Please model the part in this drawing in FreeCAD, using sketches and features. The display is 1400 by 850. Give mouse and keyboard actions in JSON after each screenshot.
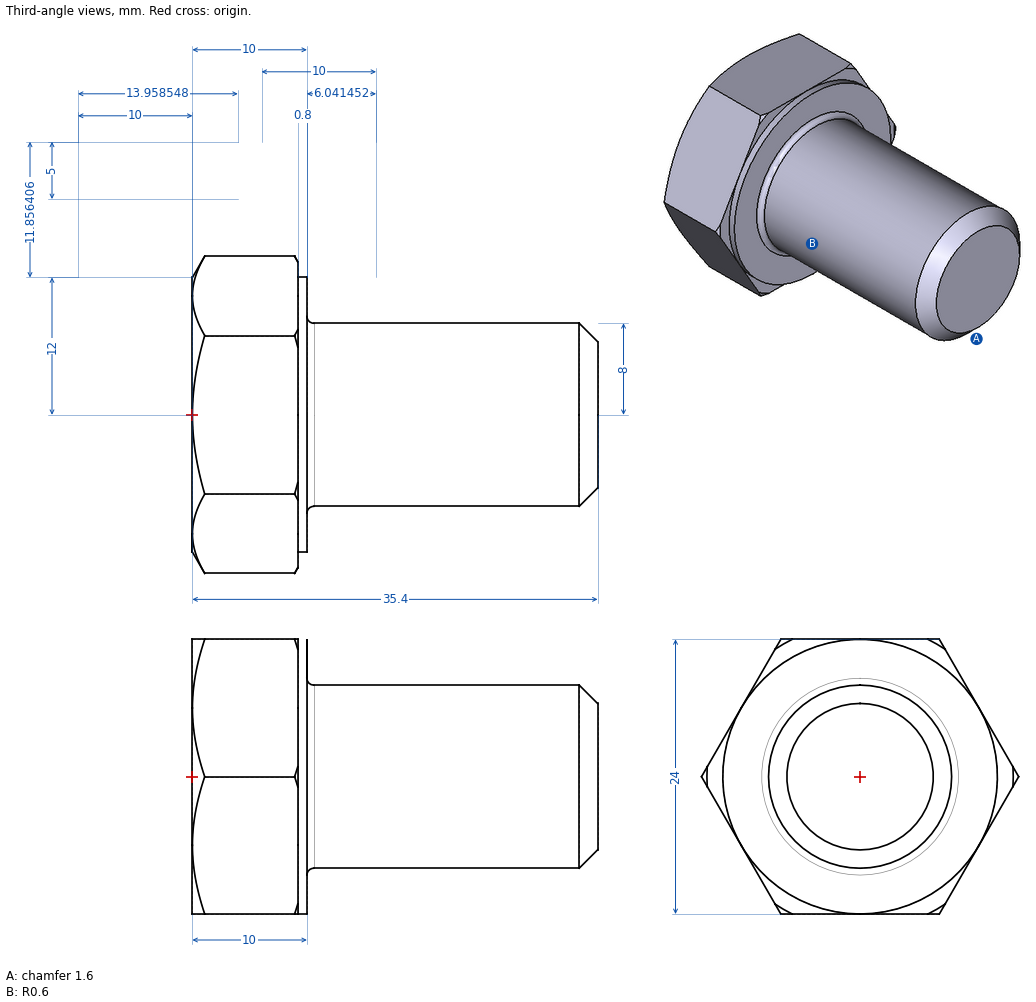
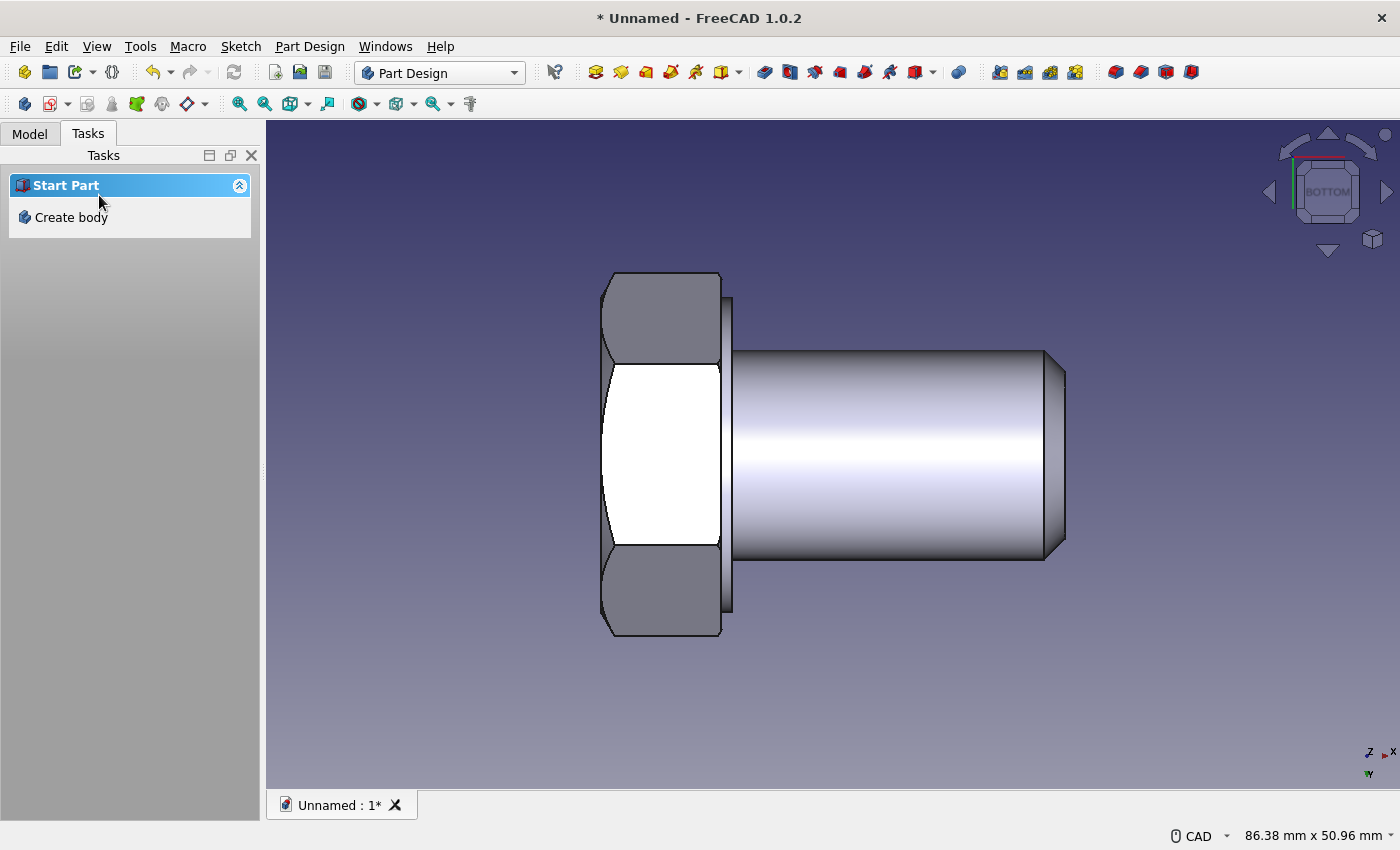
{"action": "key", "text": "4"}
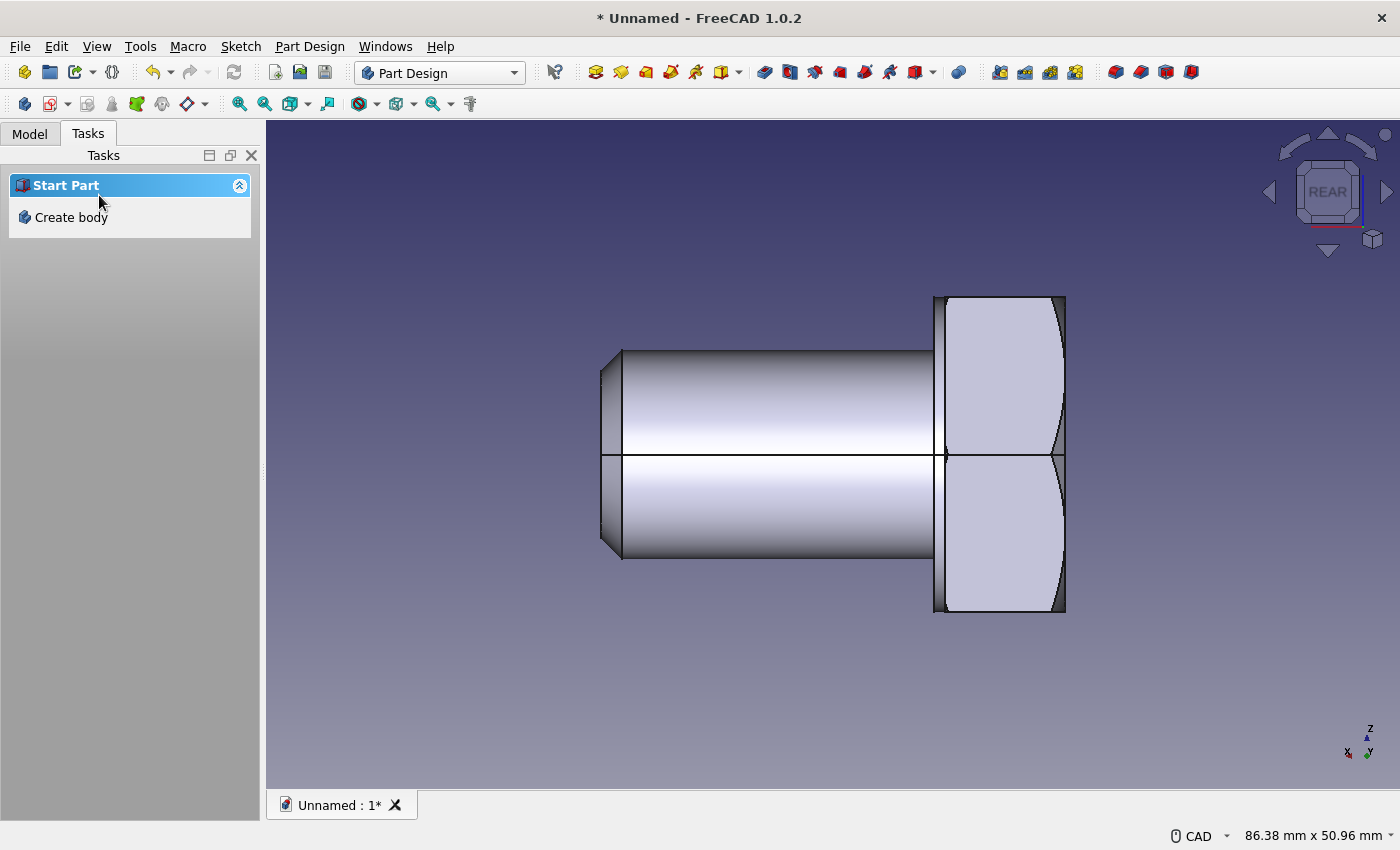
{"action": "key", "text": "6"}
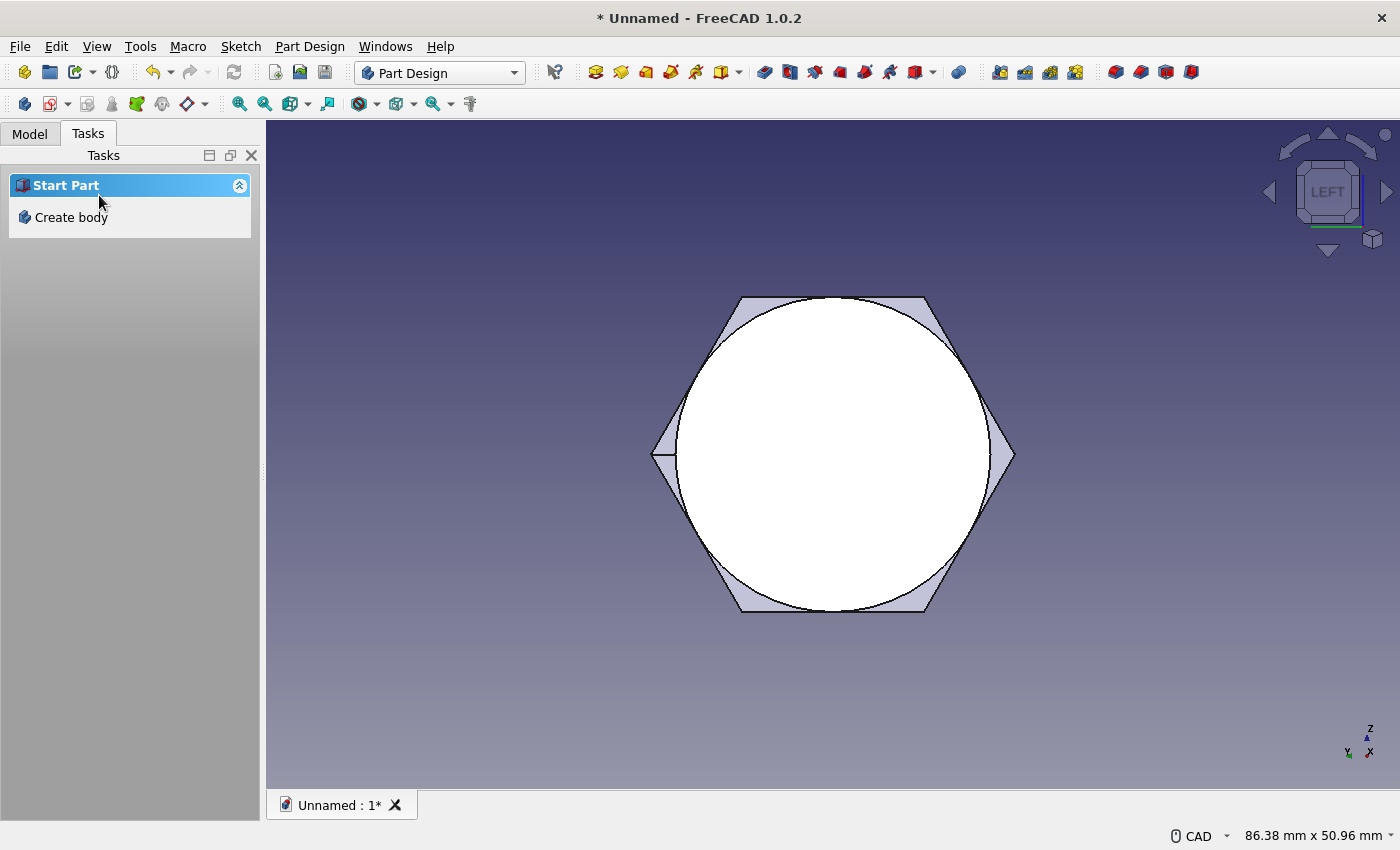
{"action": "key", "text": "v 3"}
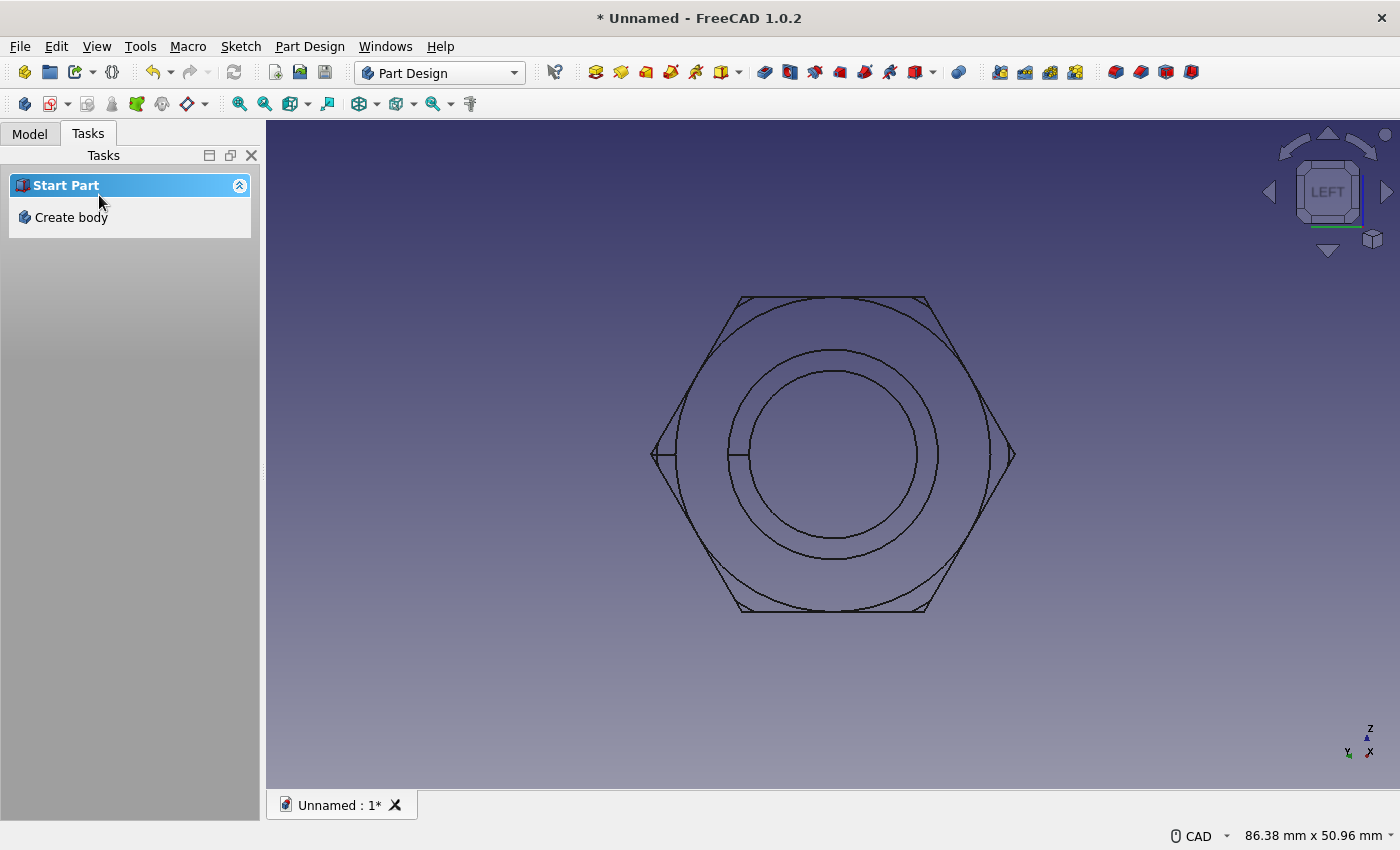
{"action": "key", "text": "0"}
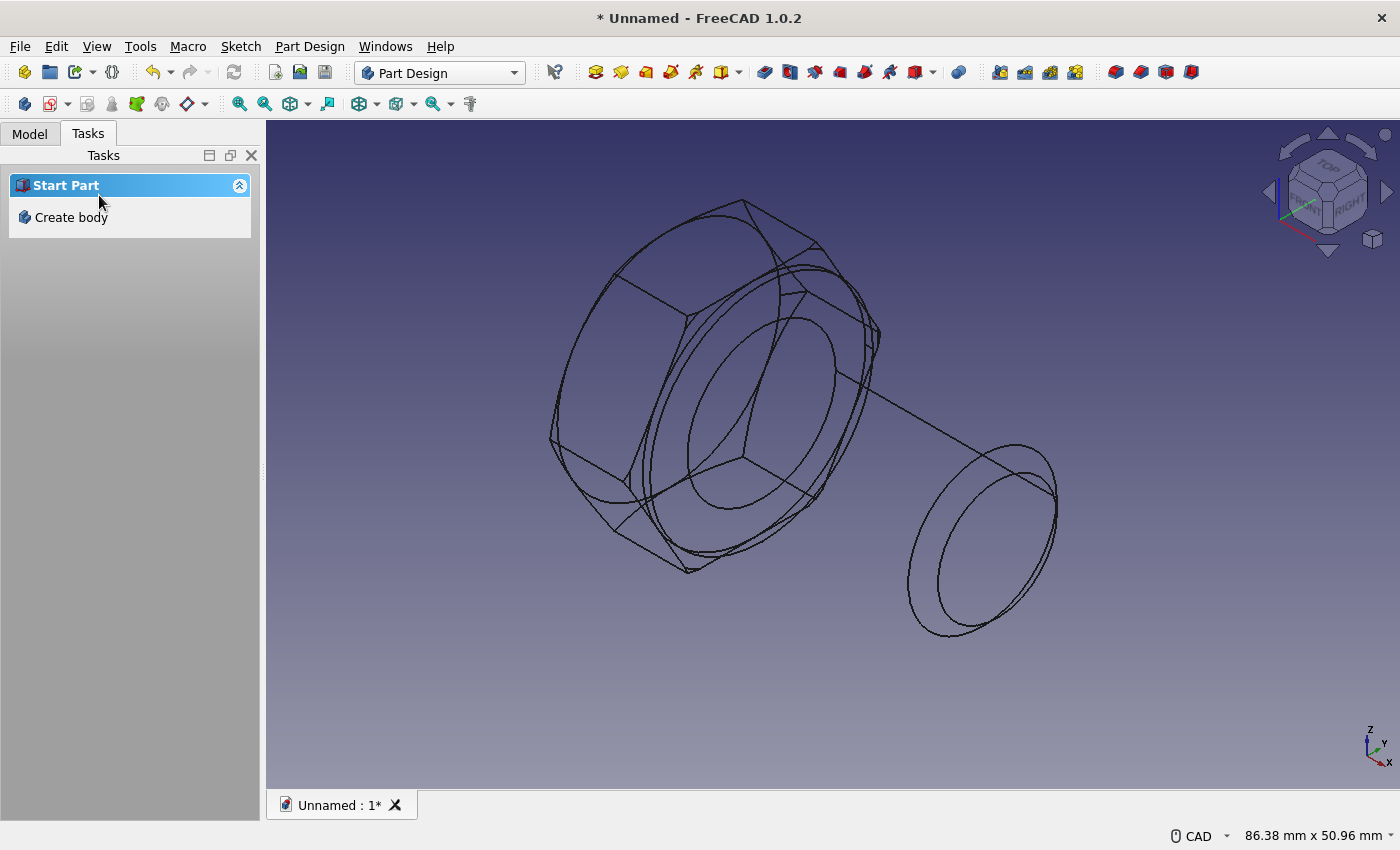
{"action": "left_click", "coordinate": [687, 455]}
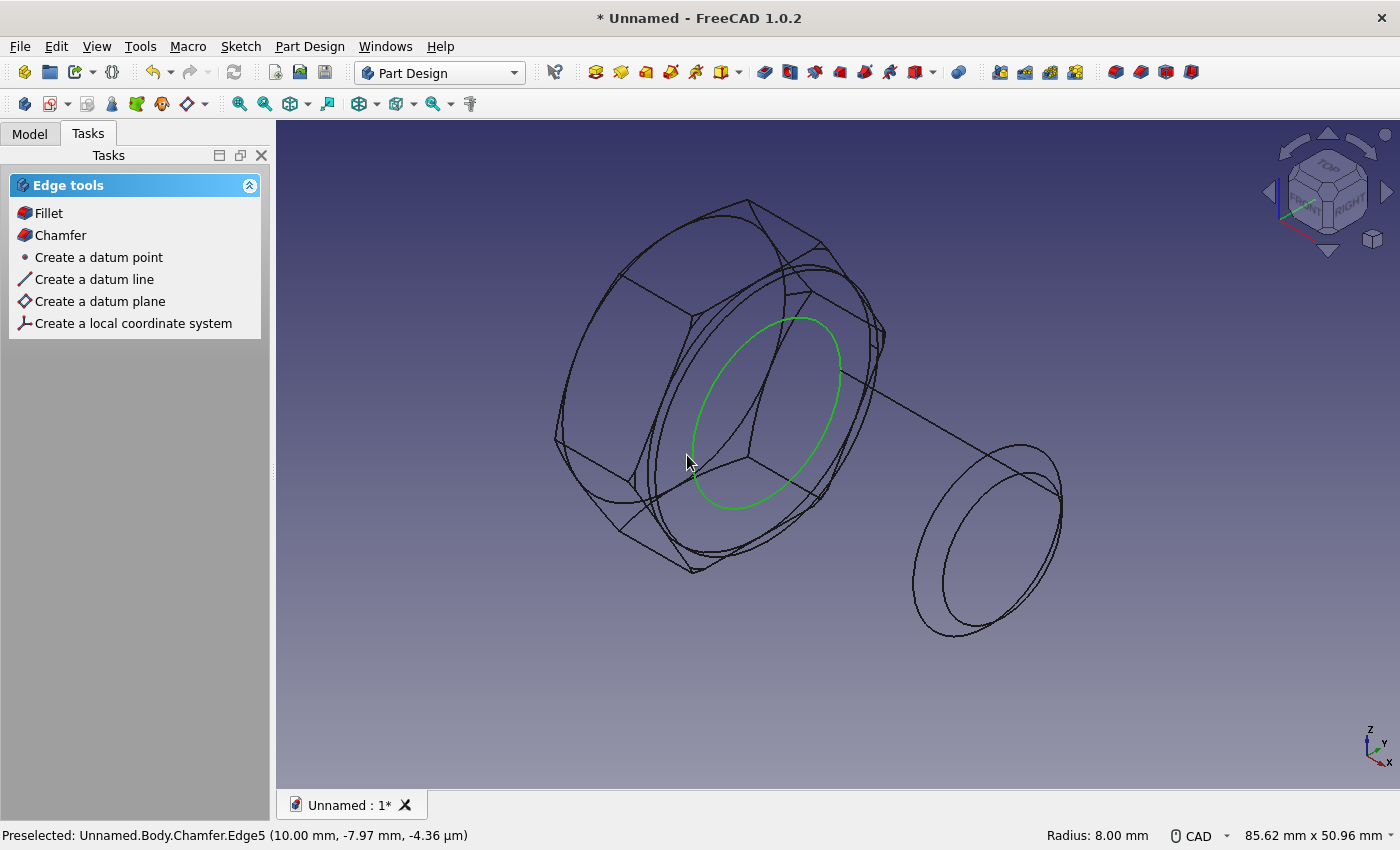
{"action": "key", "text": "v 1"}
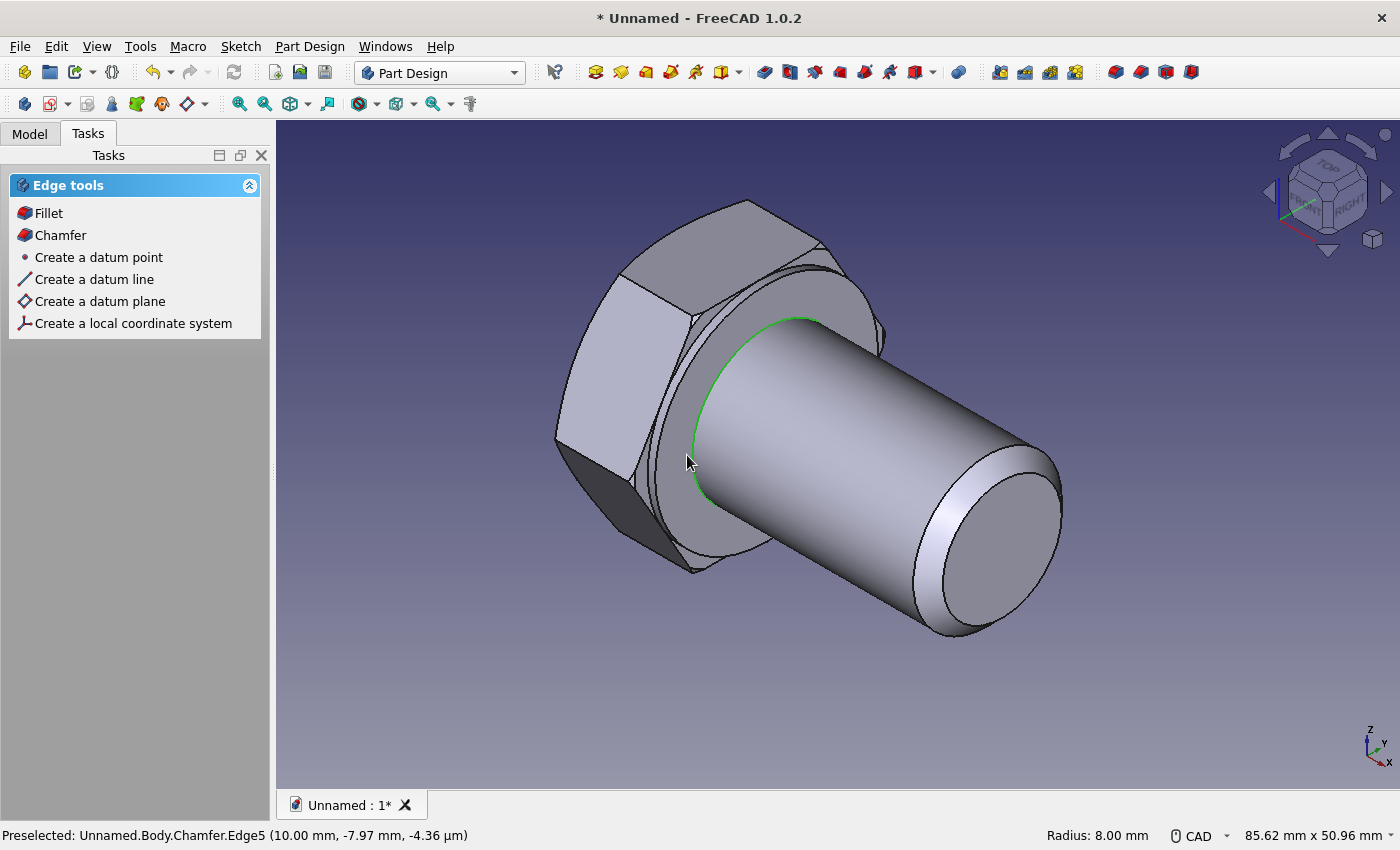
{"action": "left_click", "coordinate": [1116, 72]}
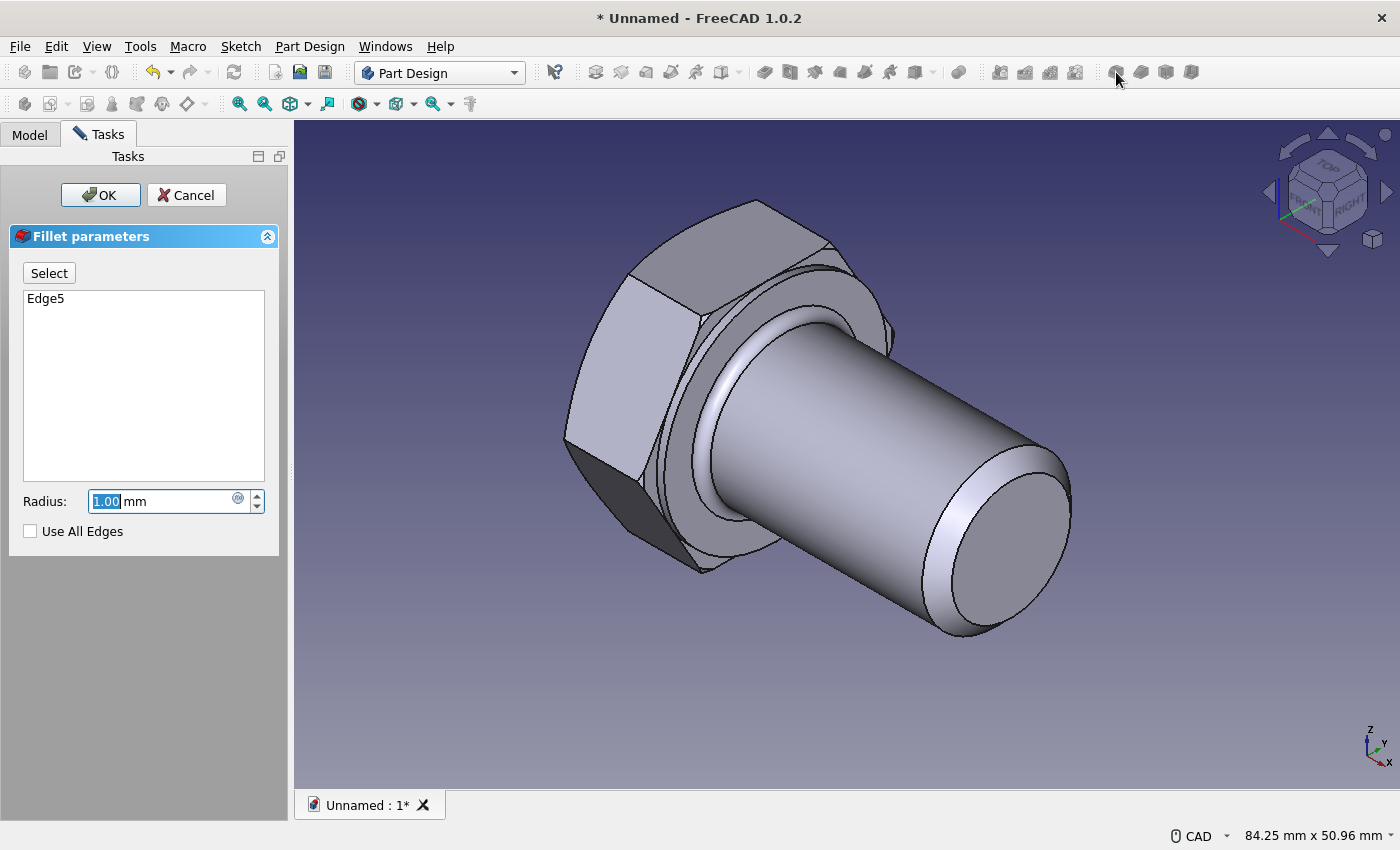
{"action": "type", "text": "0.6"}
{"action": "key", "text": "Tab"}